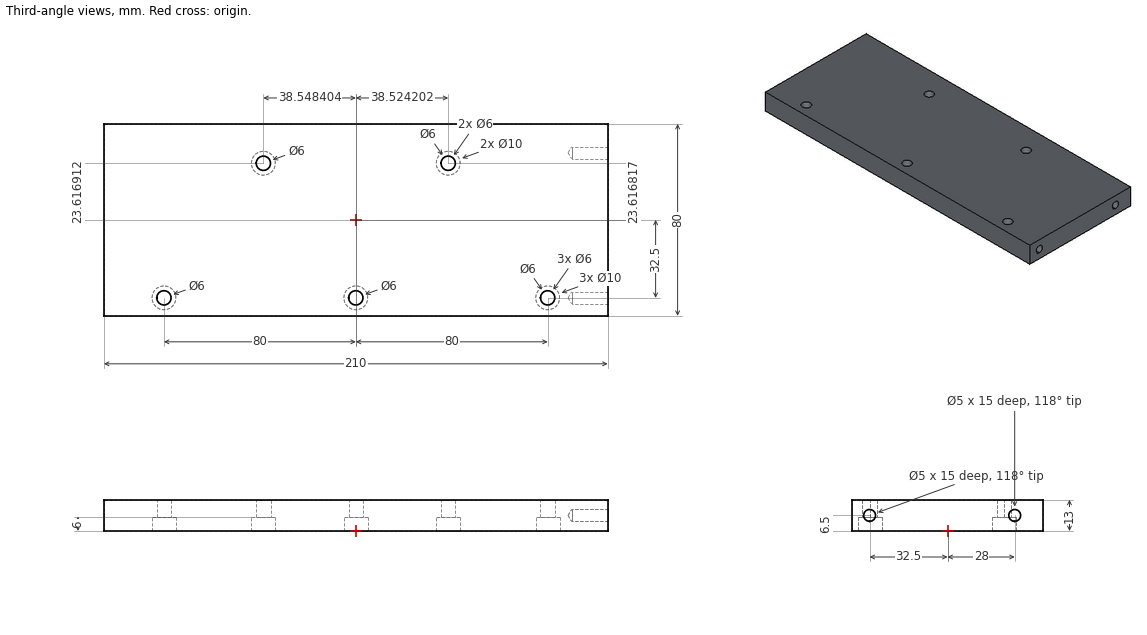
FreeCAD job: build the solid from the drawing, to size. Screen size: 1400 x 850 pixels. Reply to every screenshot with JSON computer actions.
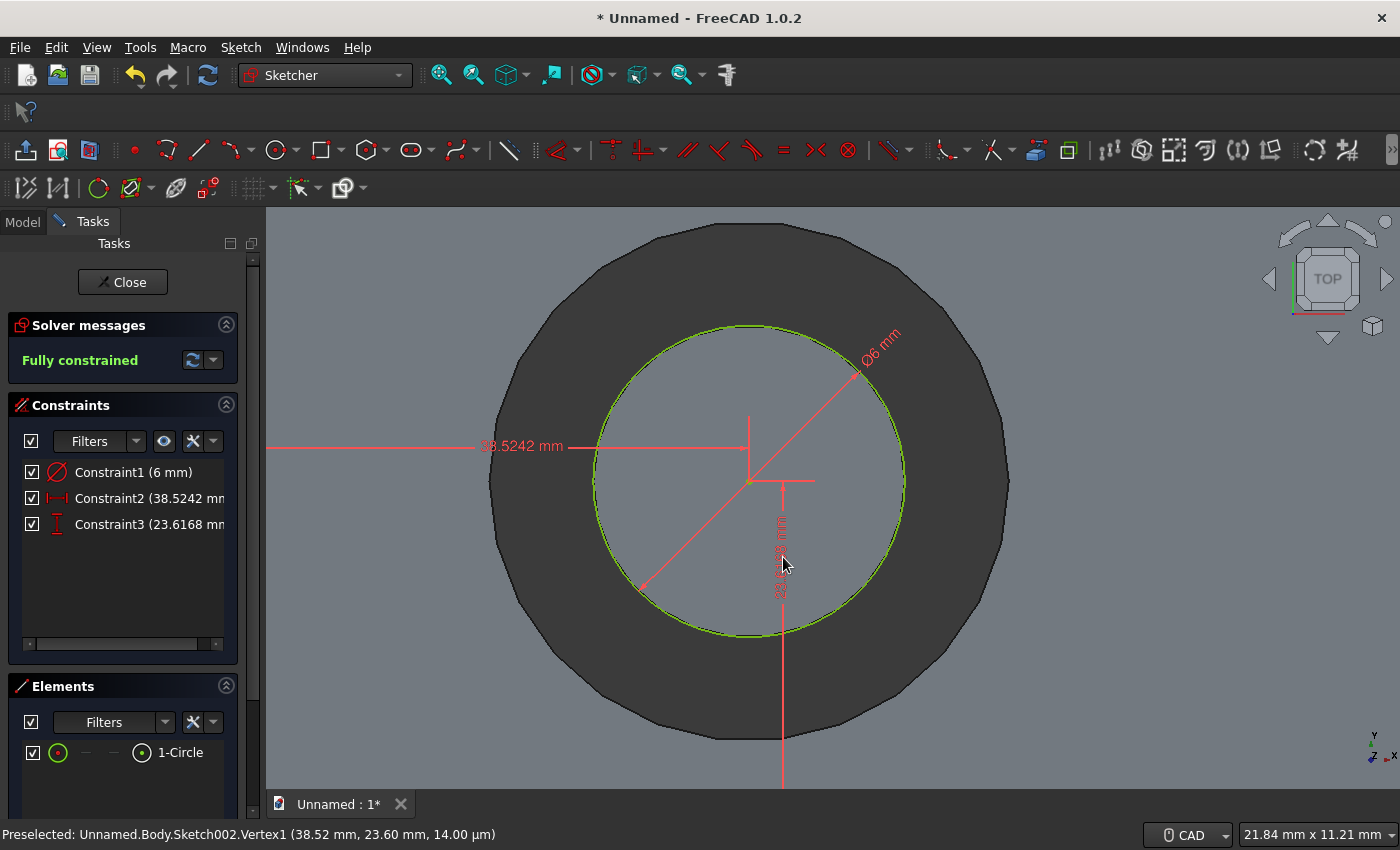
{"action": "left_click", "coordinate": [123, 282]}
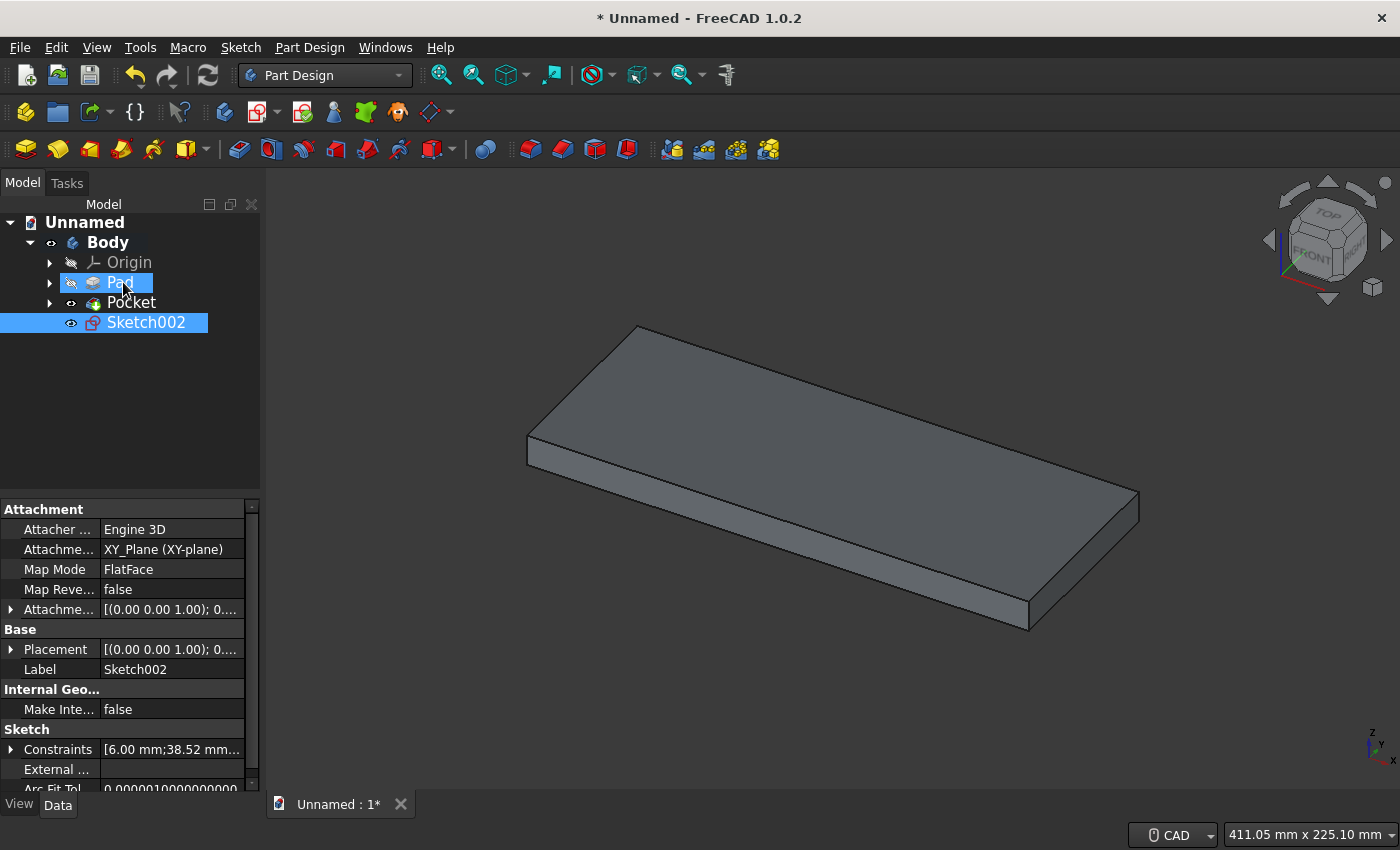
{"action": "left_click", "coordinate": [240, 150]}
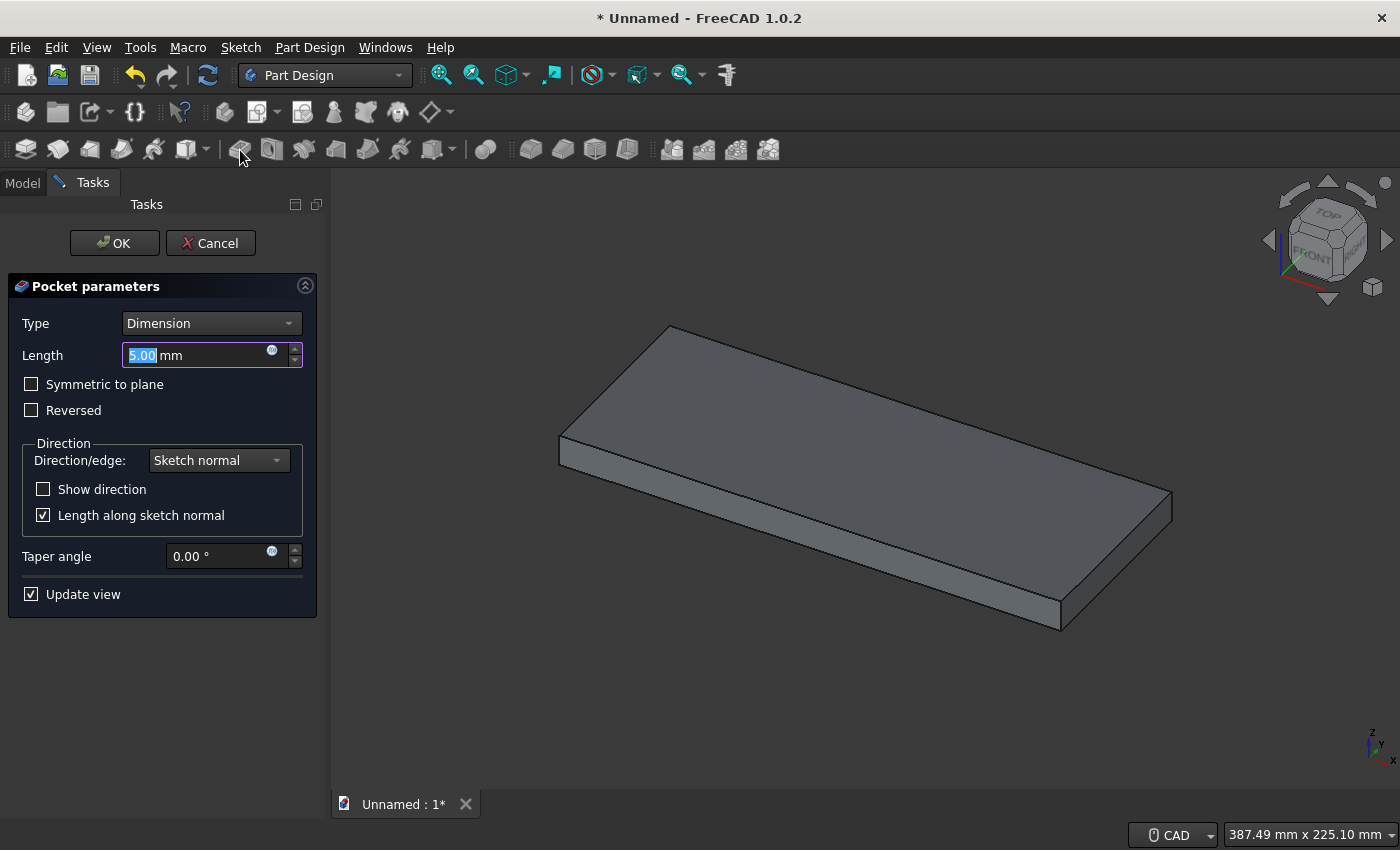
{"action": "left_click", "coordinate": [212, 324]}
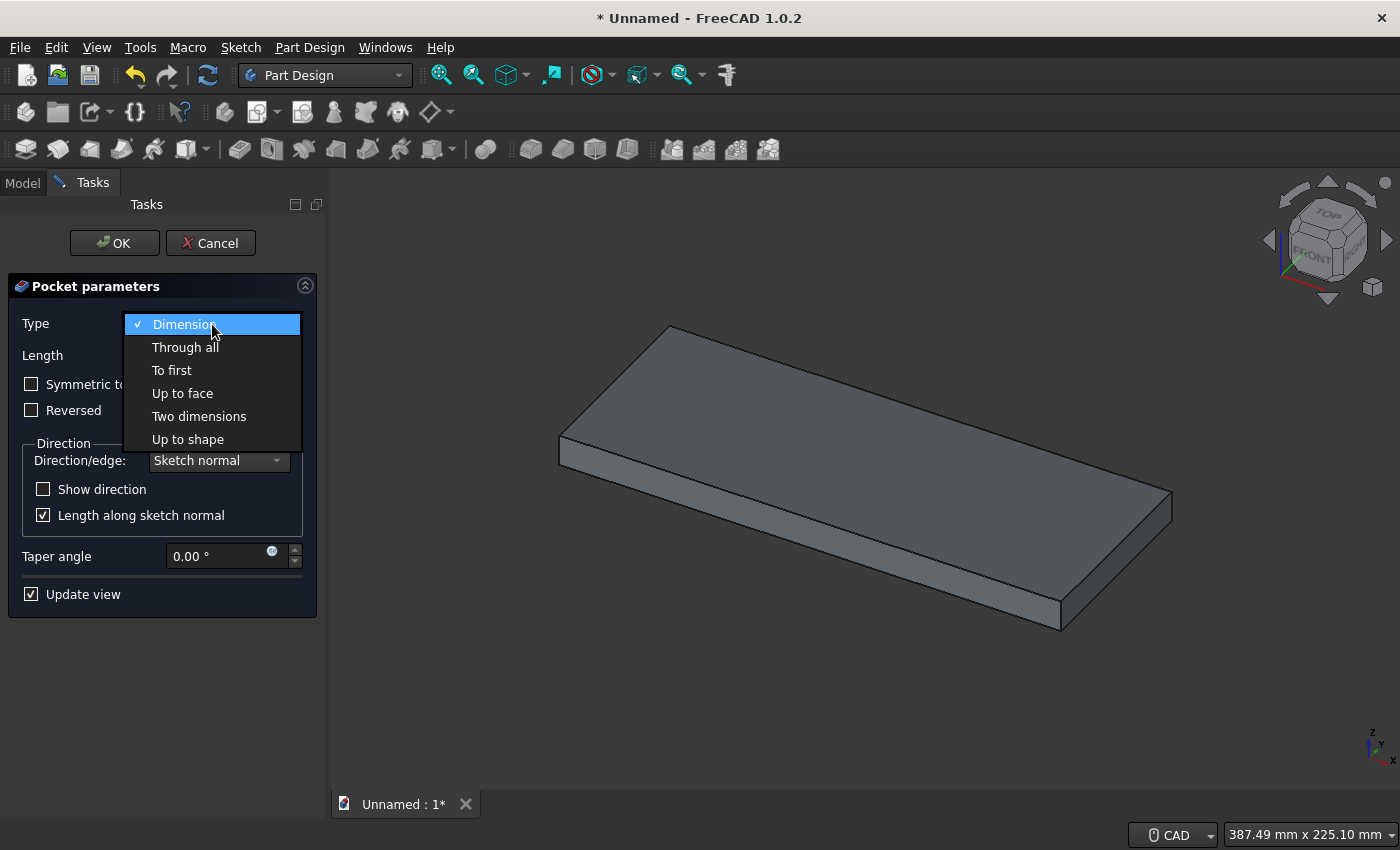
{"action": "left_click", "coordinate": [212, 370]}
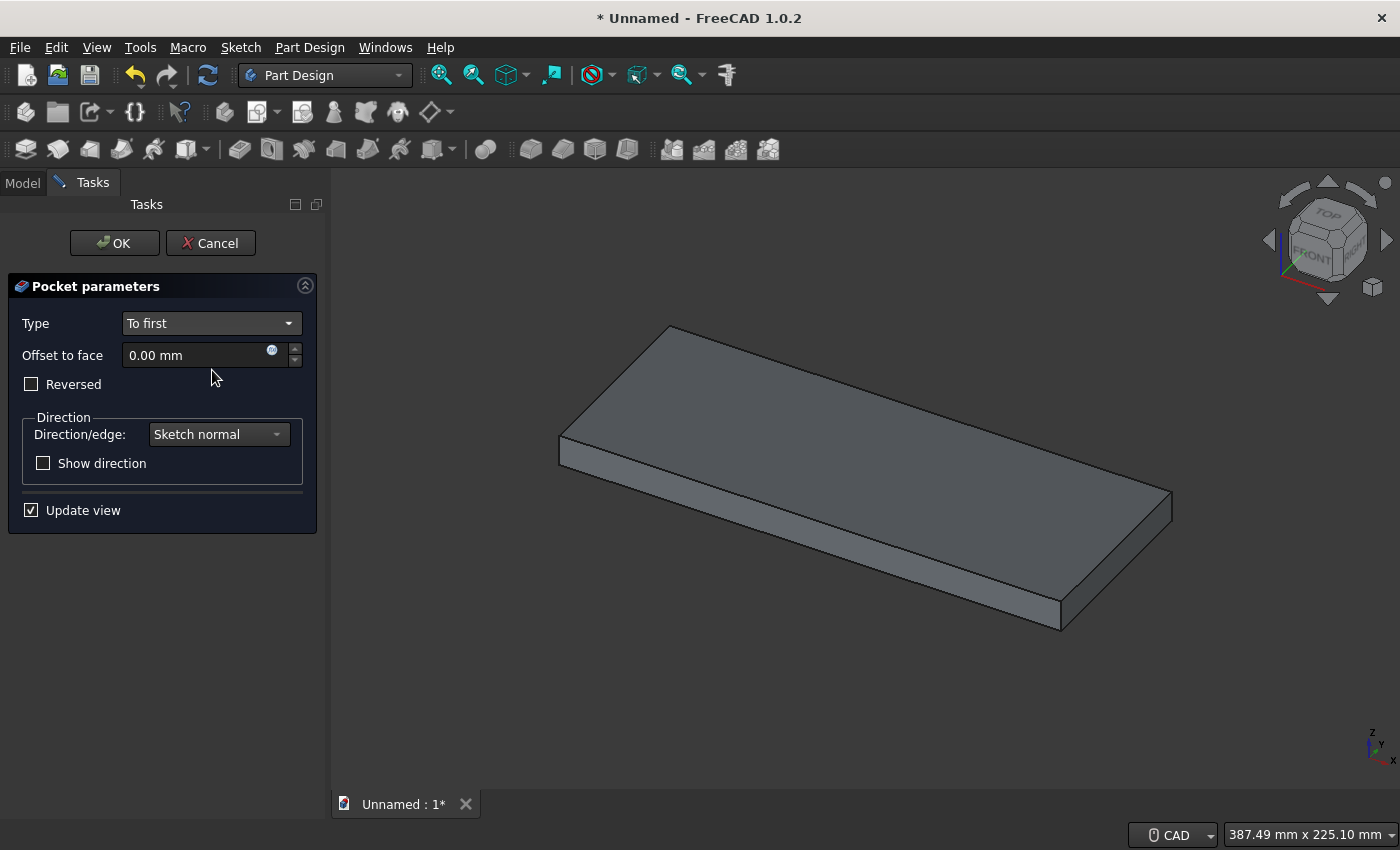
{"action": "left_click", "coordinate": [30, 384]}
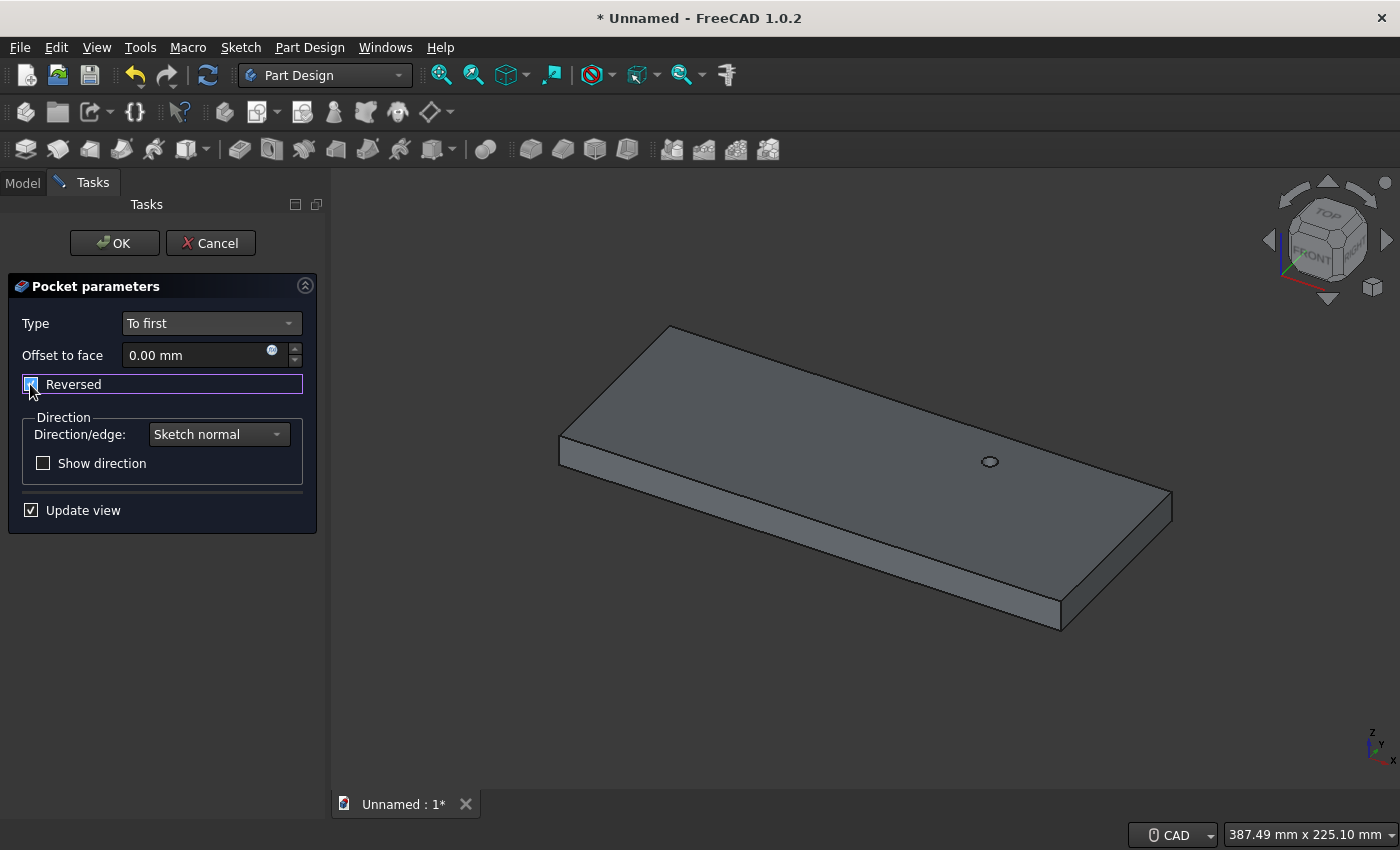
{"action": "left_click", "coordinate": [115, 243]}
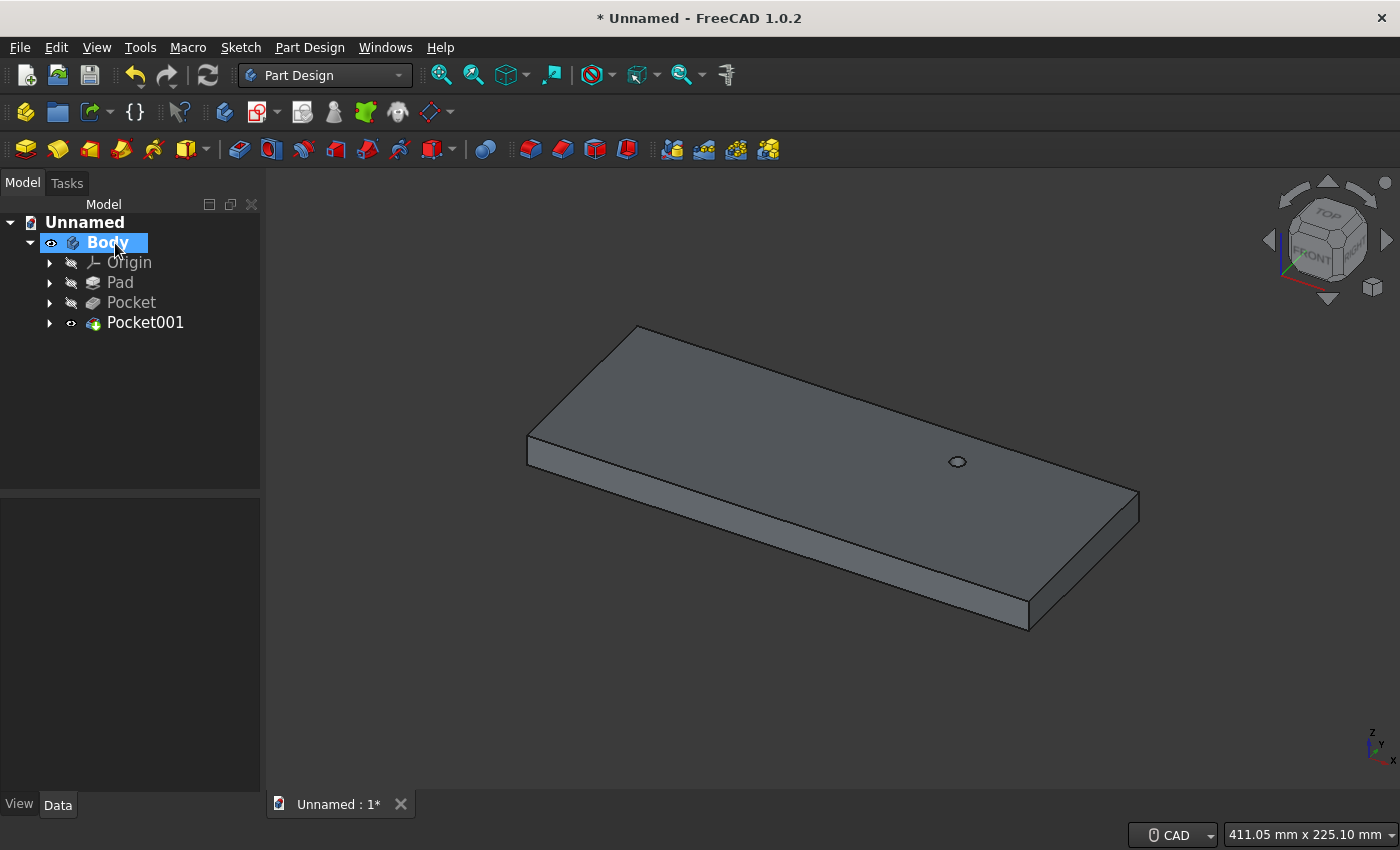
{"action": "key", "text": "5"}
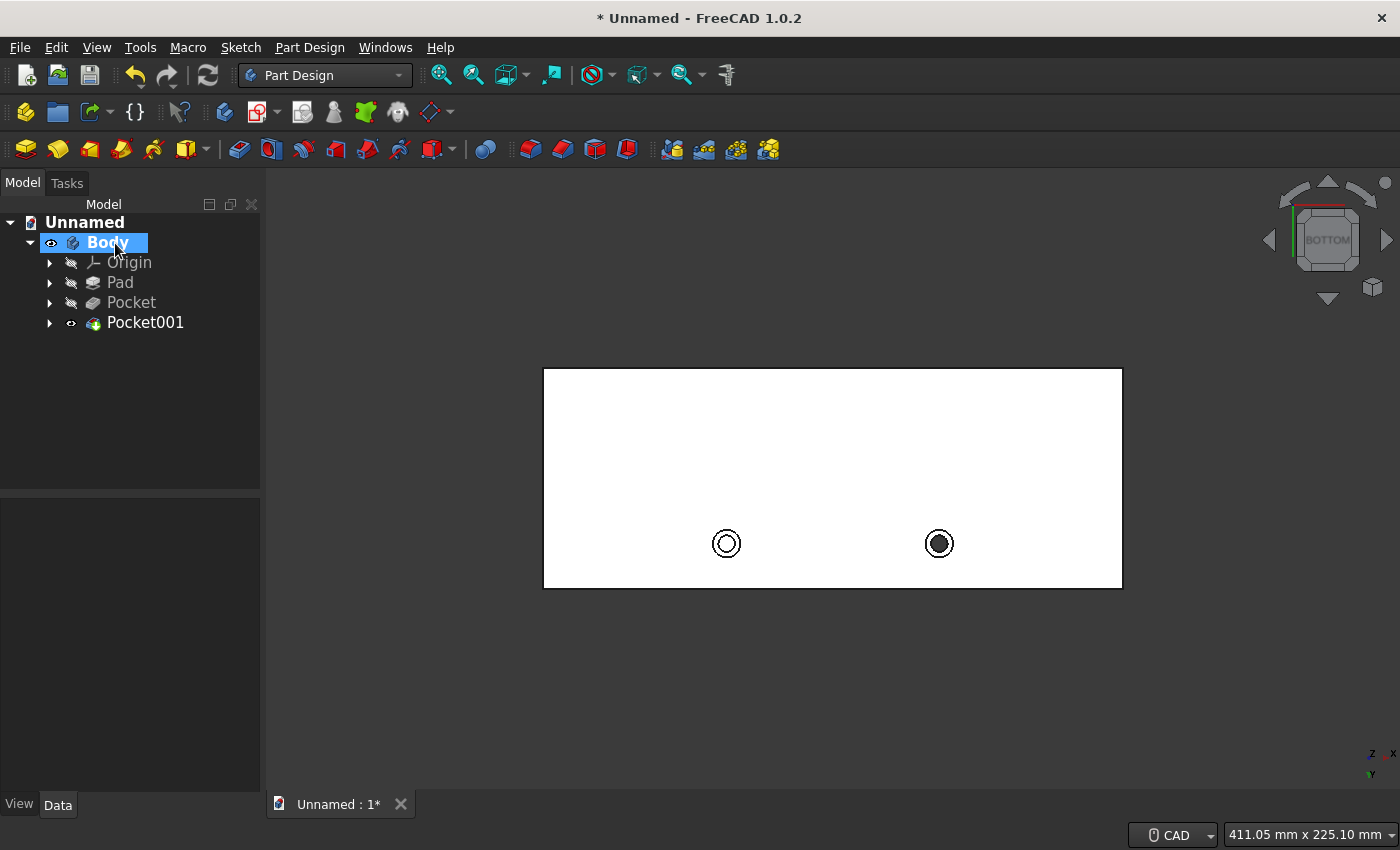
{"action": "left_click", "coordinate": [833, 477]}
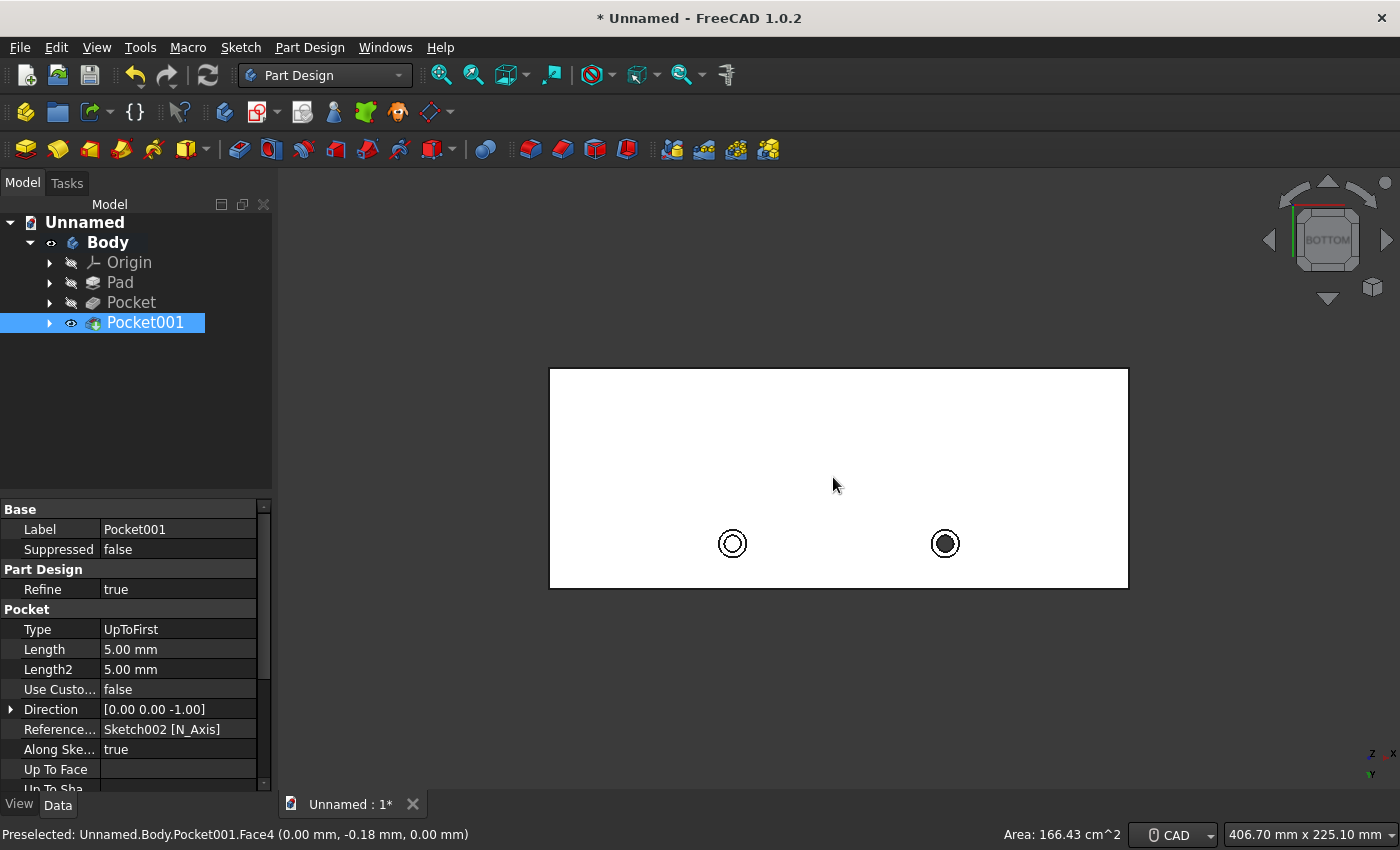
{"action": "left_click", "coordinate": [258, 112]}